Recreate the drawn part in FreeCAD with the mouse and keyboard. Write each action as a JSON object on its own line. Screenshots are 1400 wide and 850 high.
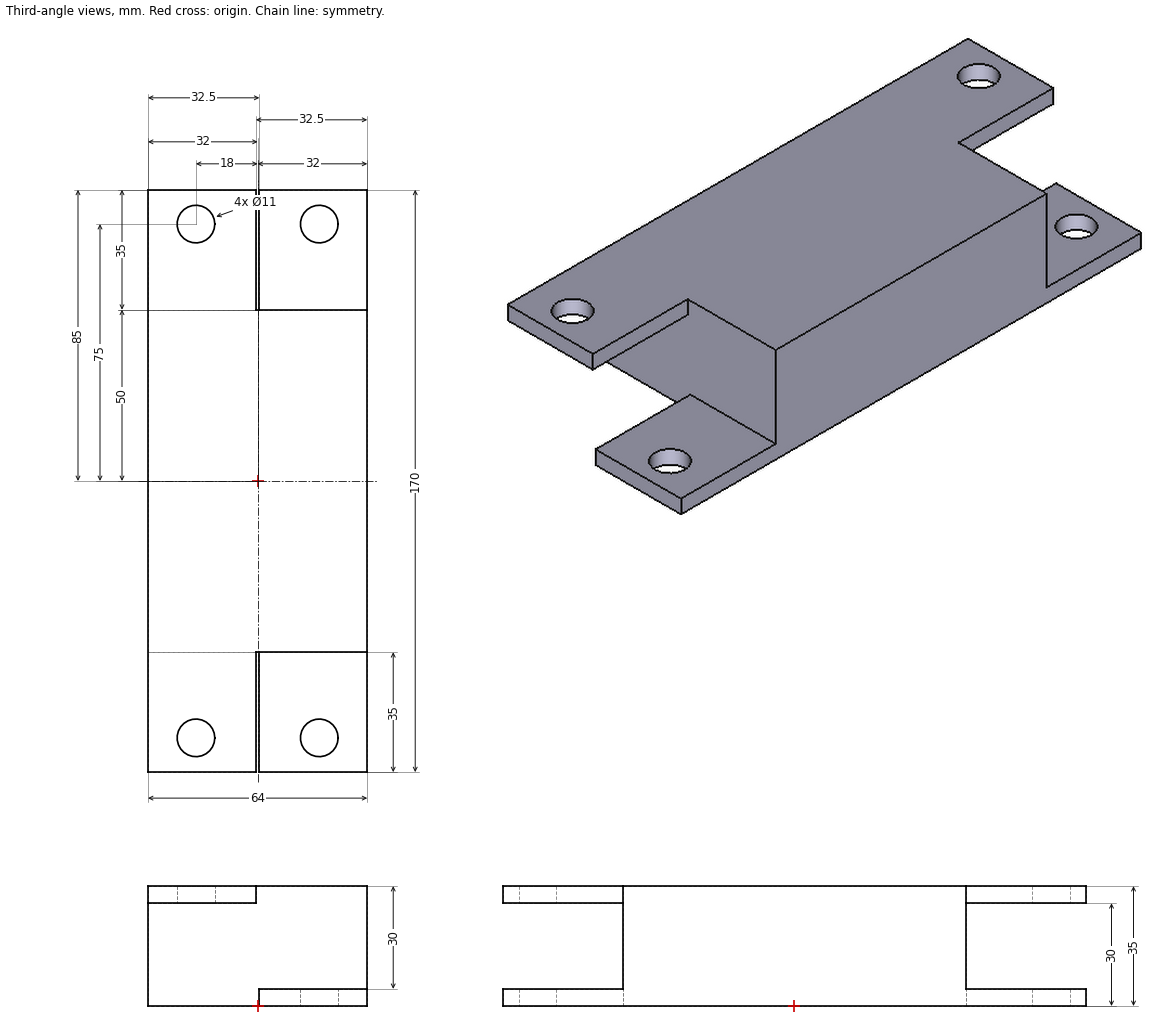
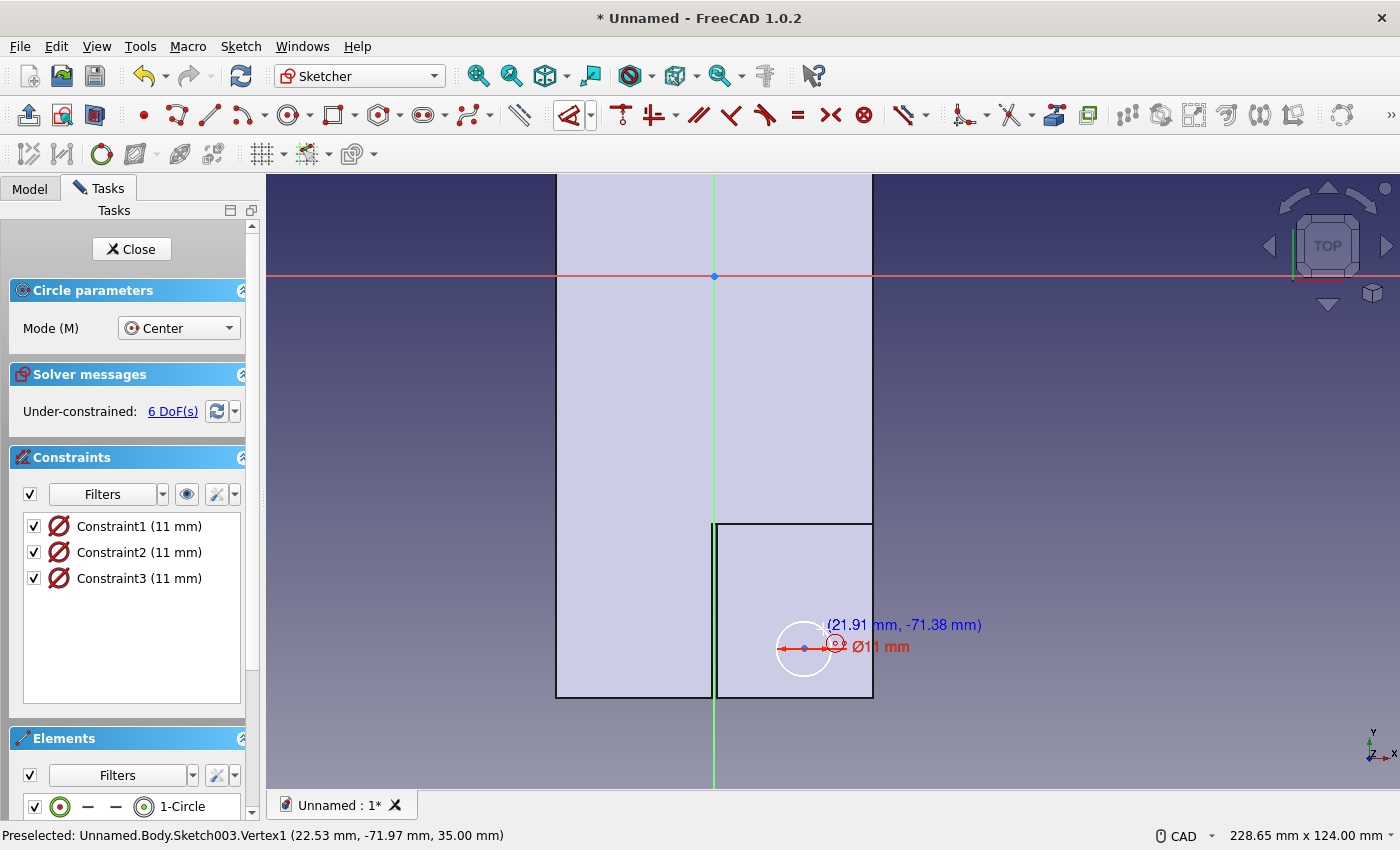
{"action": "left_click", "coordinate": [625, 648]}
{"action": "mouse_move", "coordinate": [644, 629]}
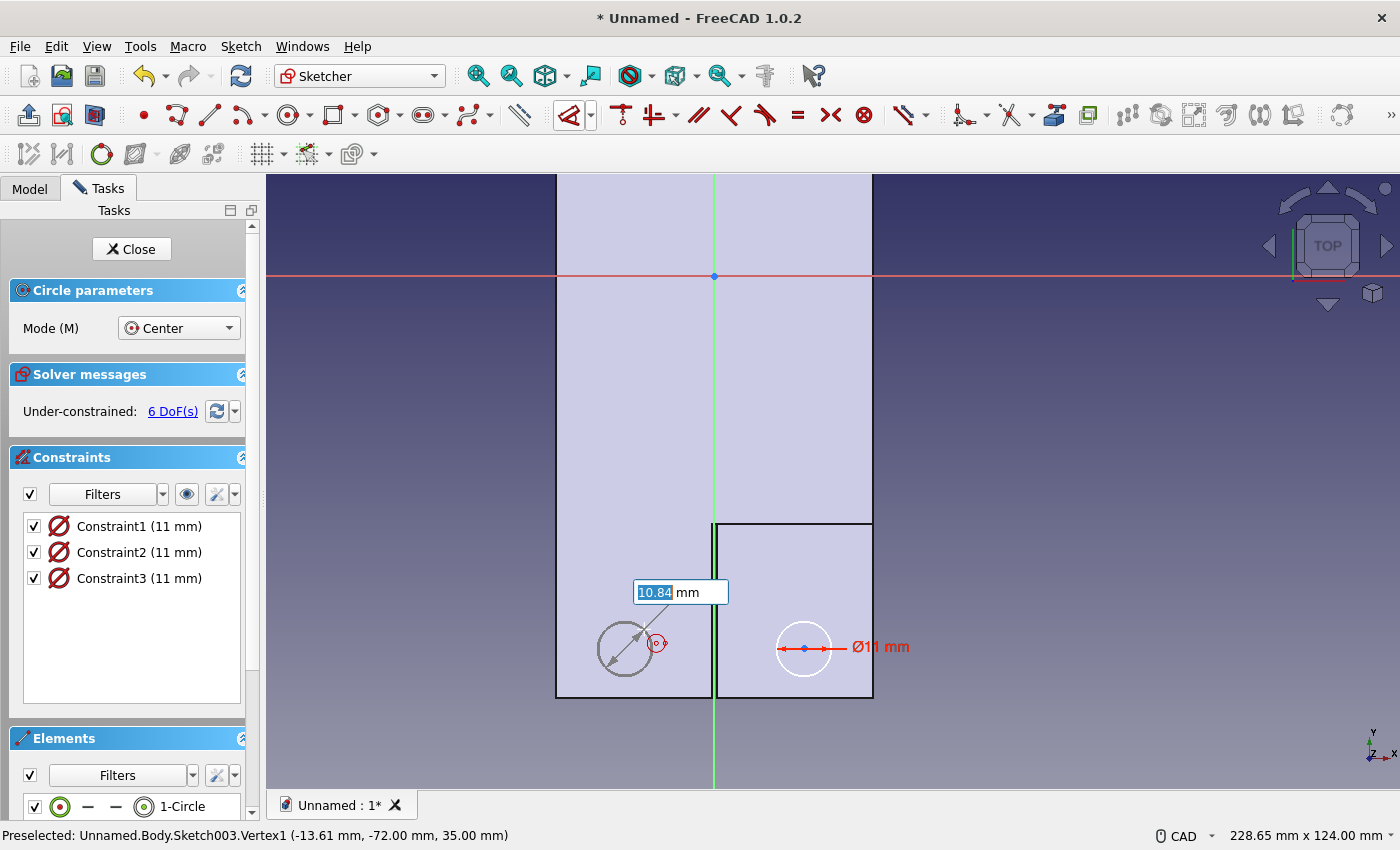
{"action": "type", "text": "11"}
{"action": "key", "text": "Return"}
{"action": "key", "text": "Escape"}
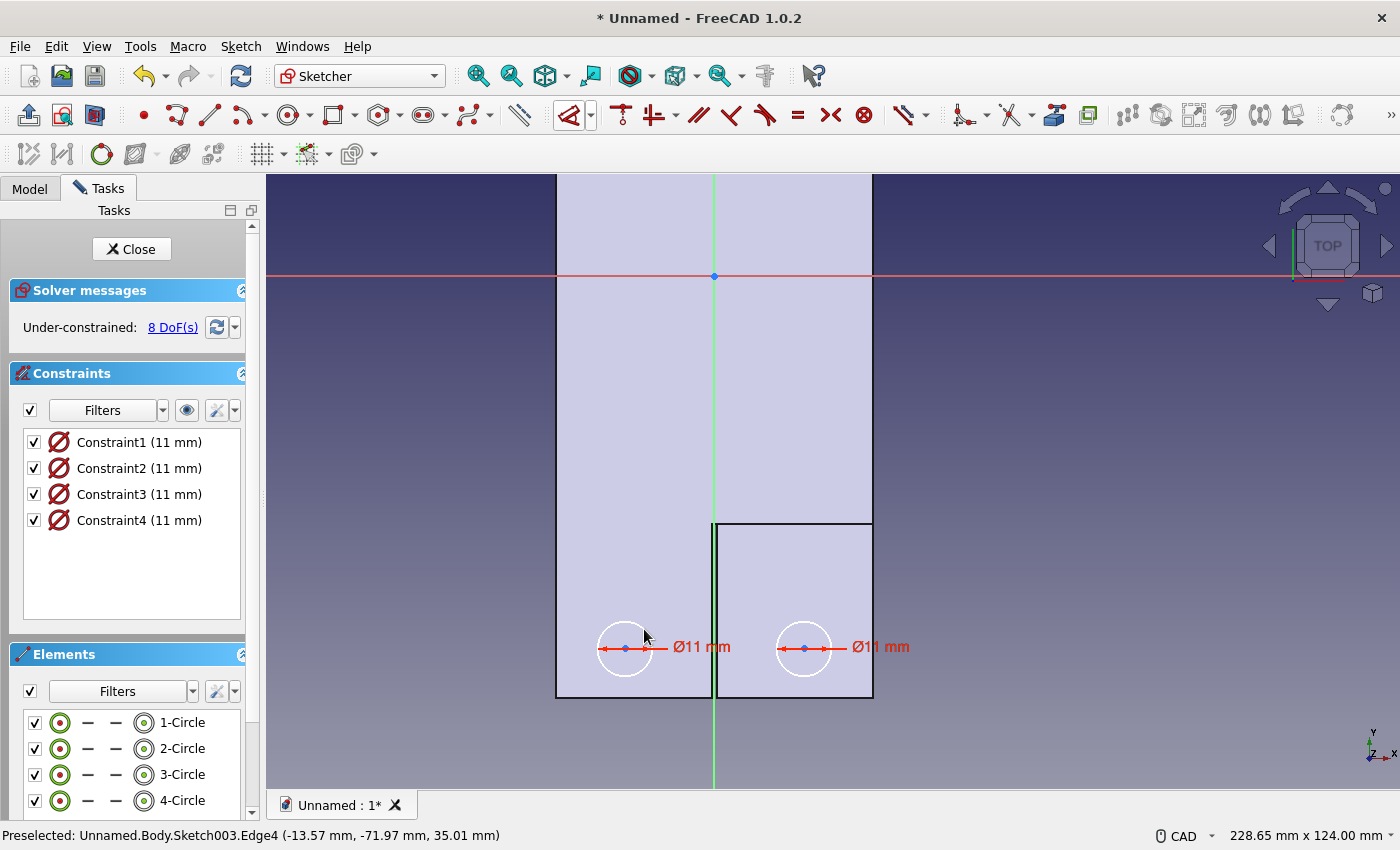
{"action": "scroll", "coordinate": [805, 649], "scroll_direction": "down", "scroll_amount": 4}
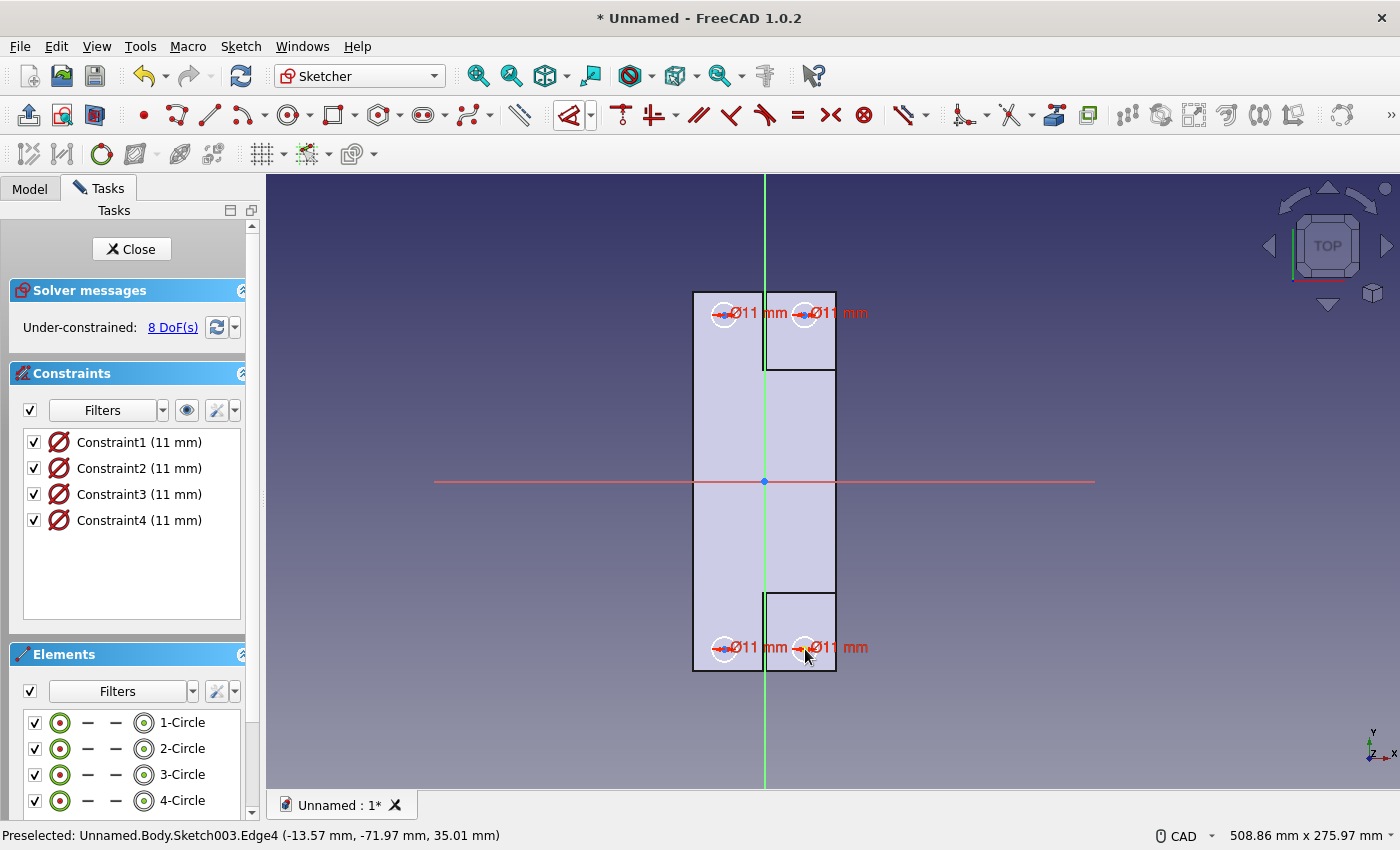
{"action": "left_click", "coordinate": [724, 315]}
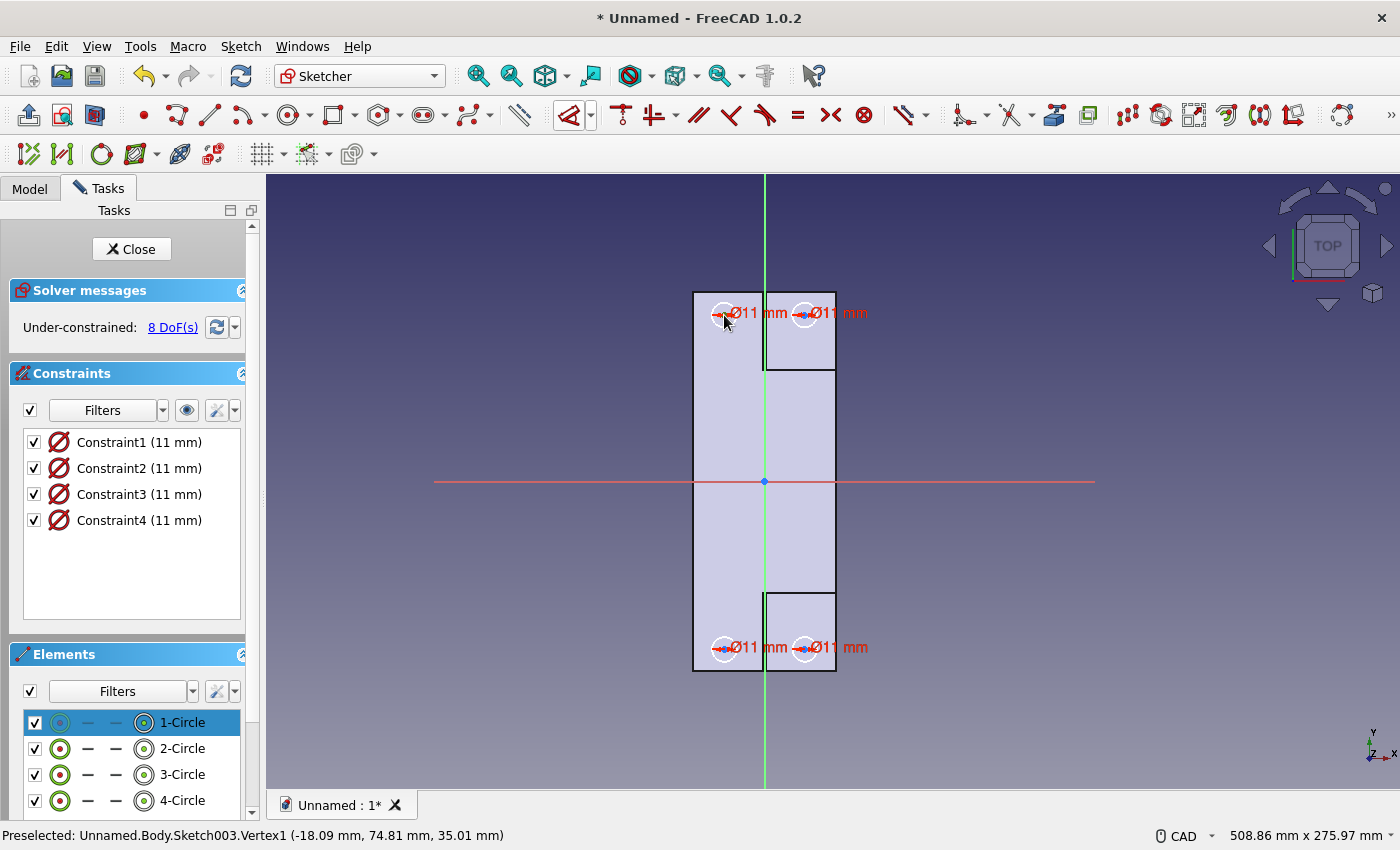
{"action": "left_click", "coordinate": [805, 315]}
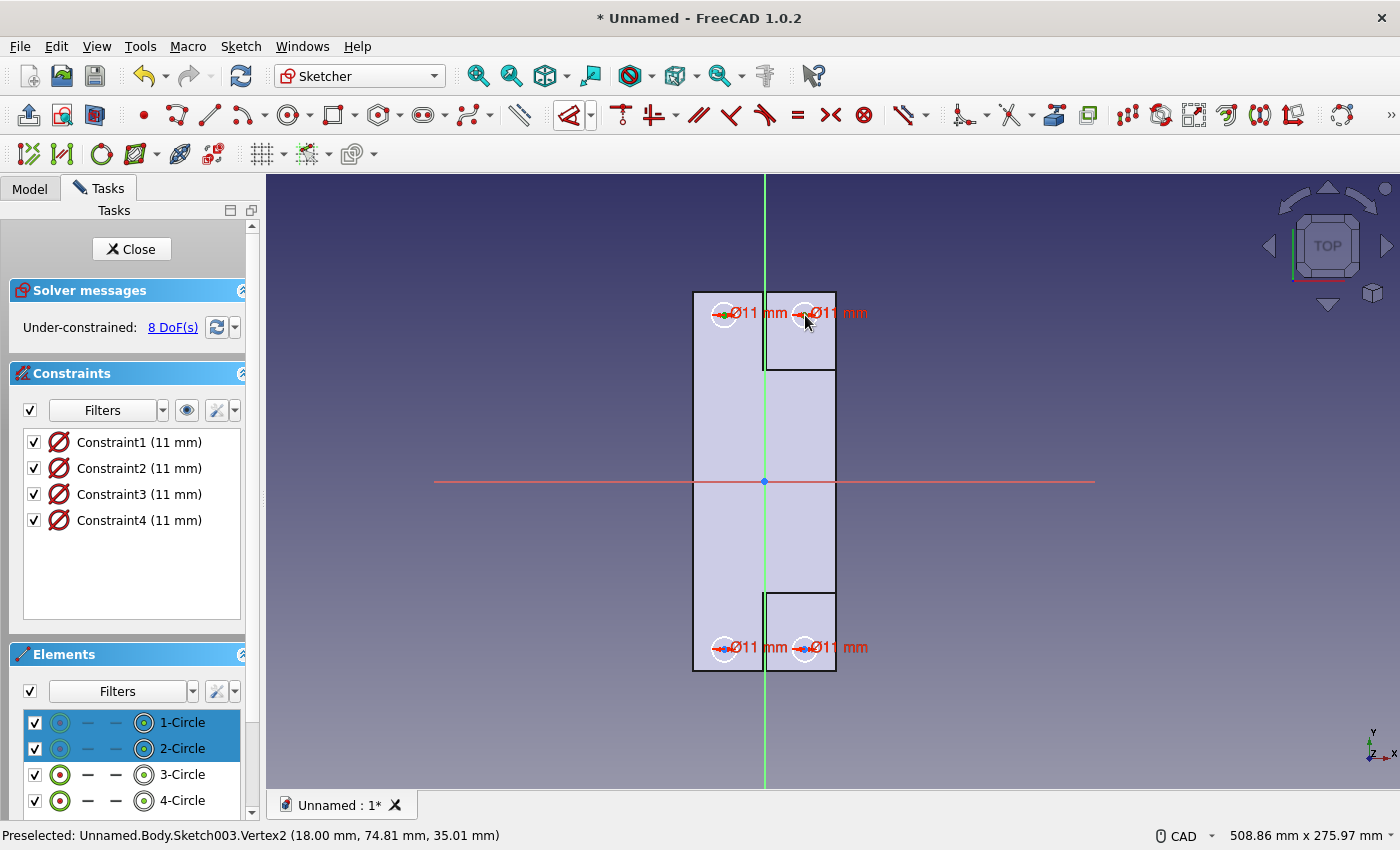
{"action": "left_click", "coordinate": [765, 721]}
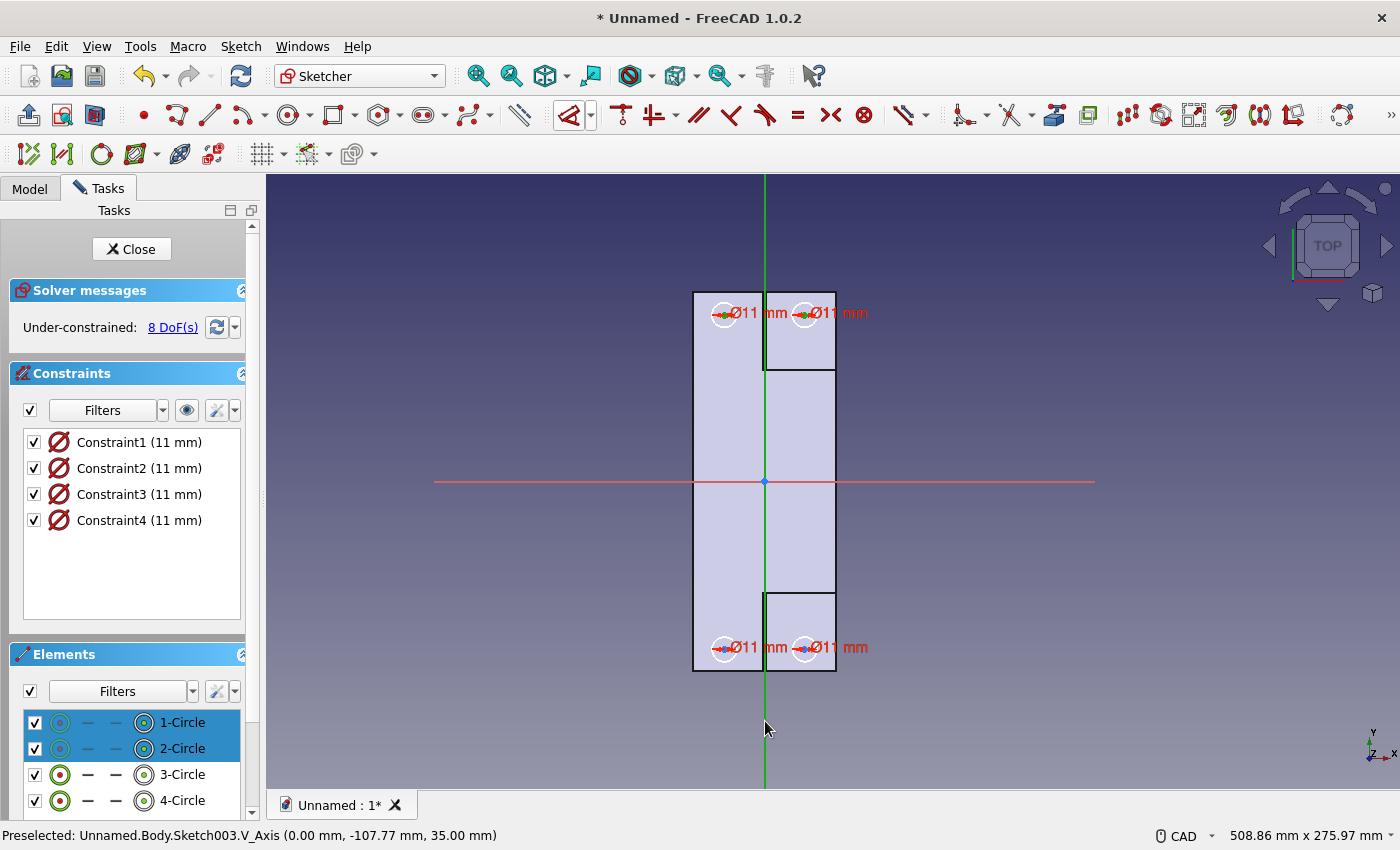
{"action": "left_click", "coordinate": [831, 116]}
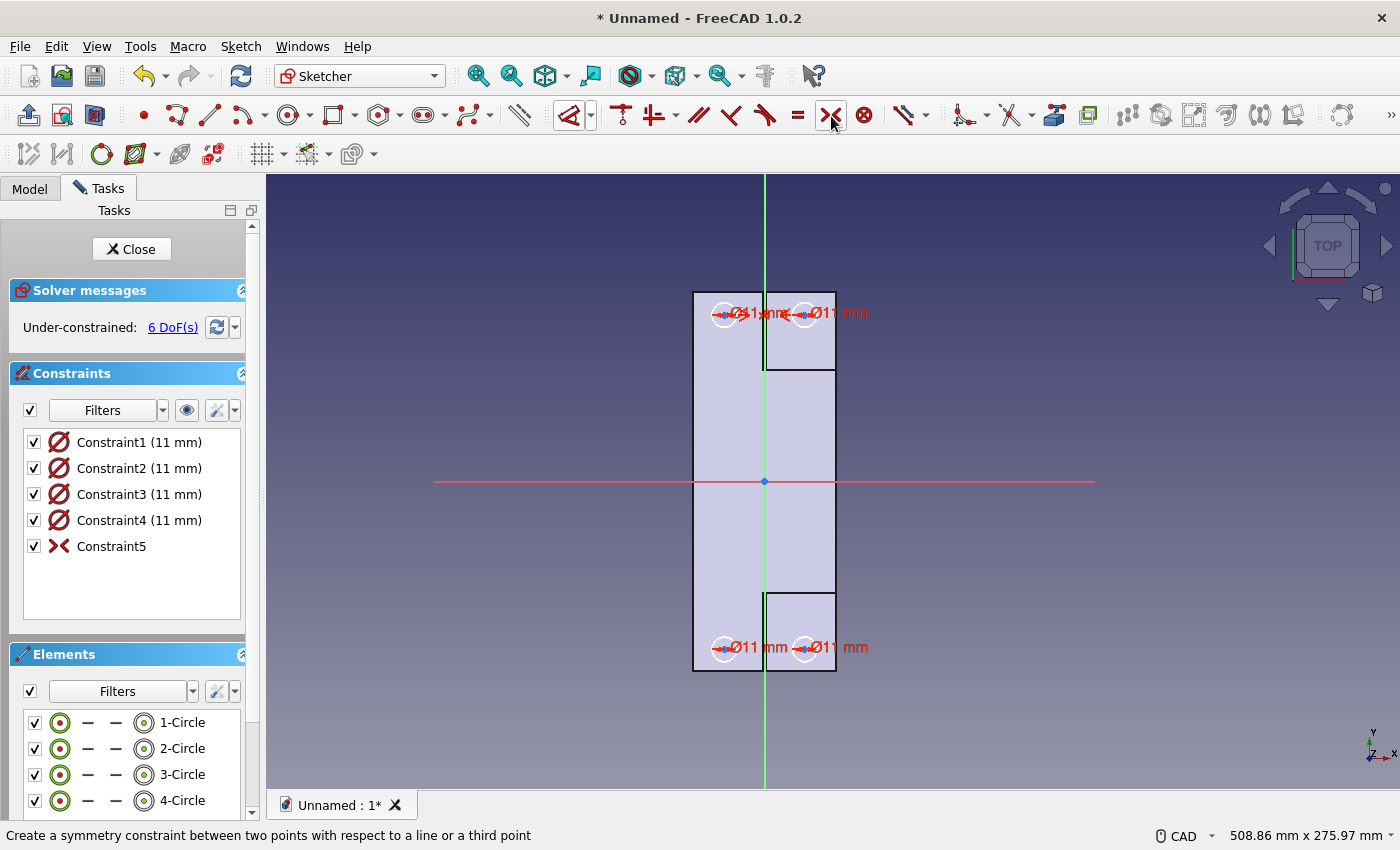
{"action": "left_click", "coordinate": [805, 315]}